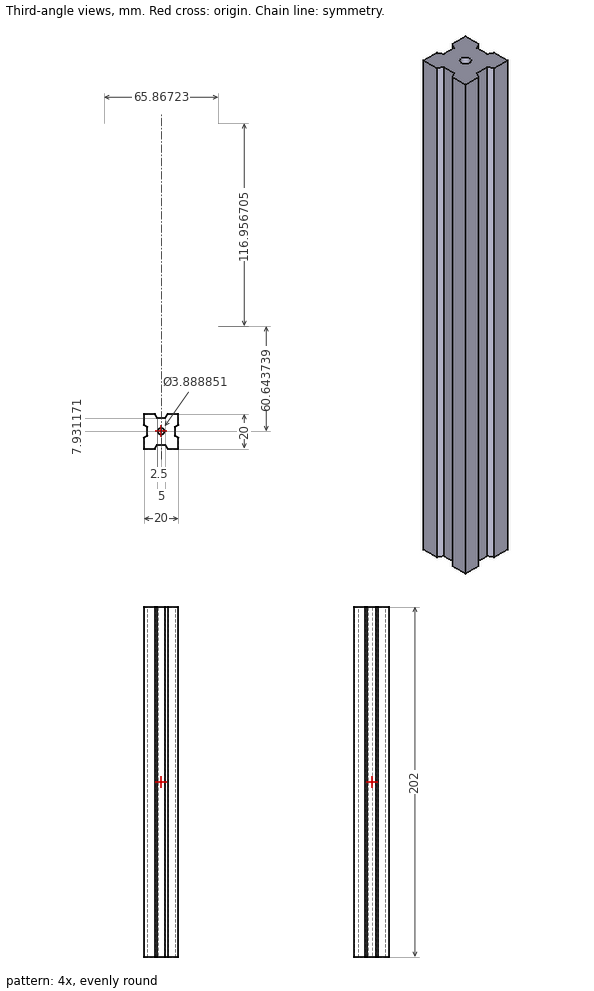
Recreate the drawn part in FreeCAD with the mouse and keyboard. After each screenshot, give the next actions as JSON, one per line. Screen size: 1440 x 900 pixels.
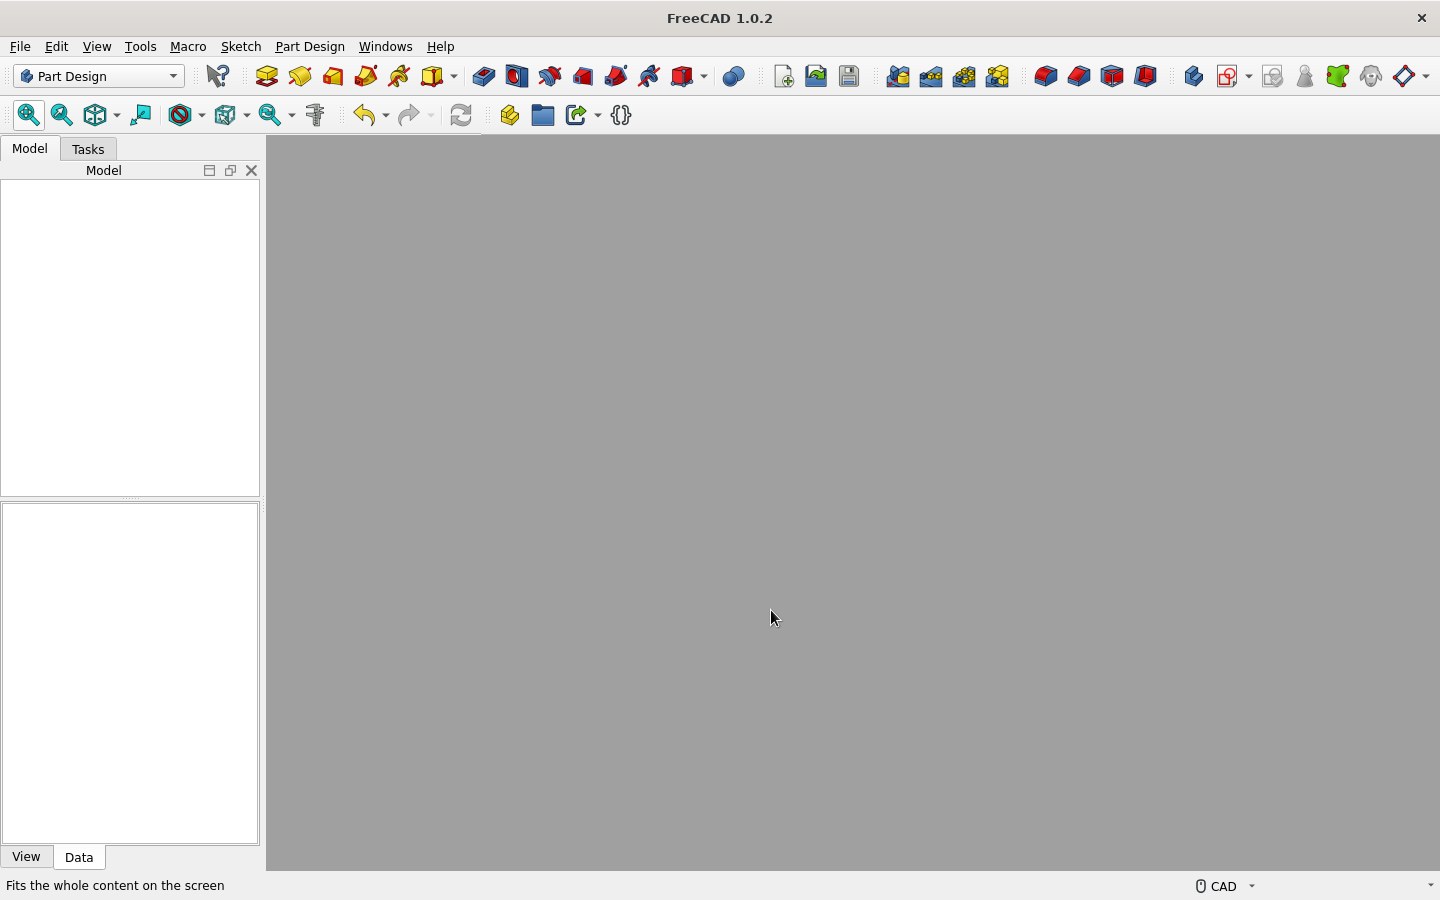
{"action": "key", "text": "ctrl+n"}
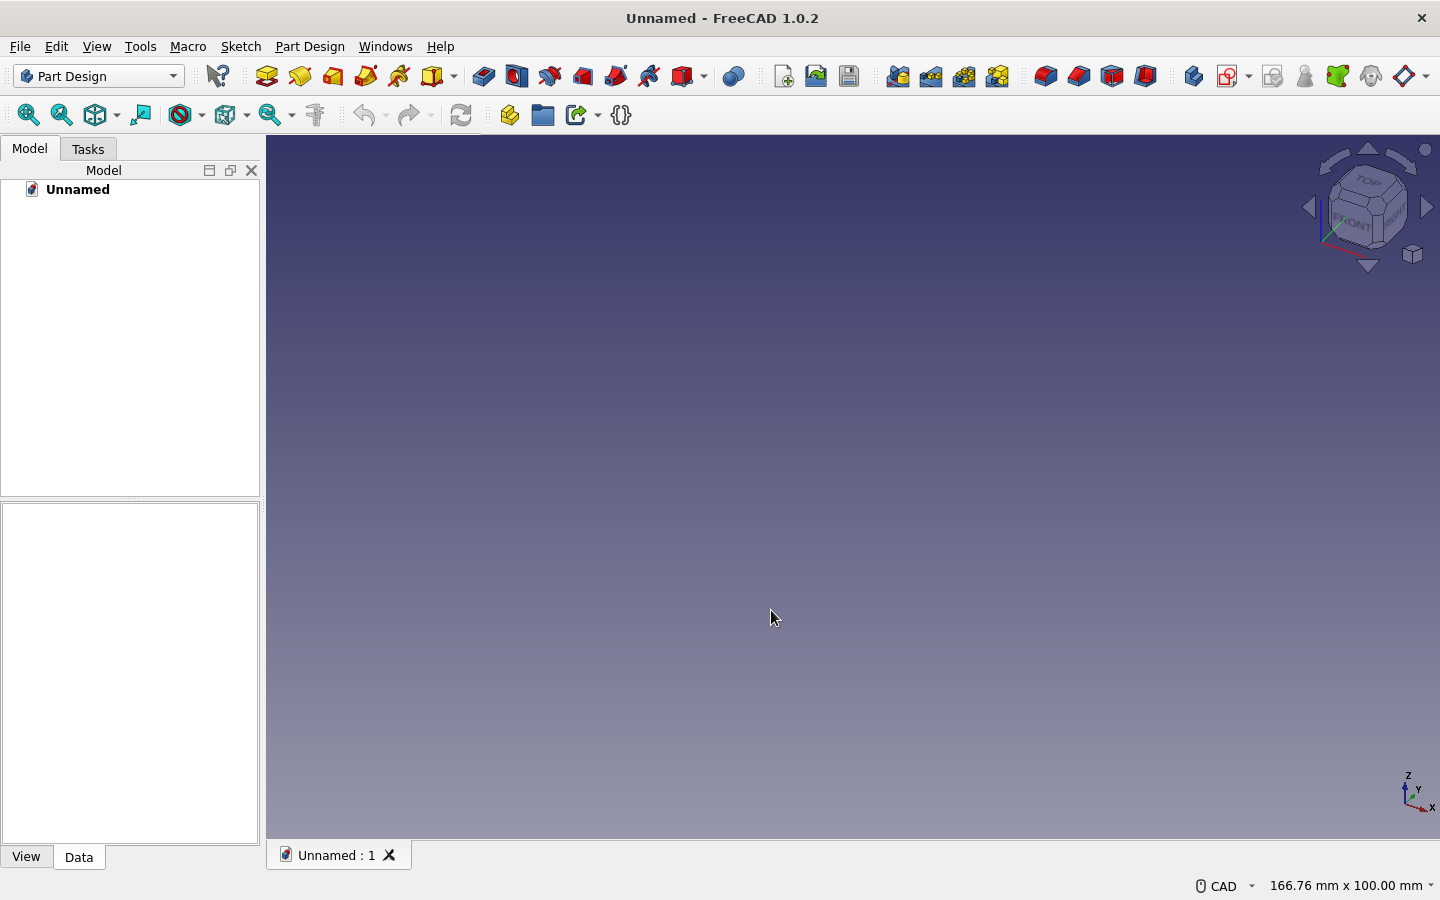
{"action": "left_click", "coordinate": [1226, 76]}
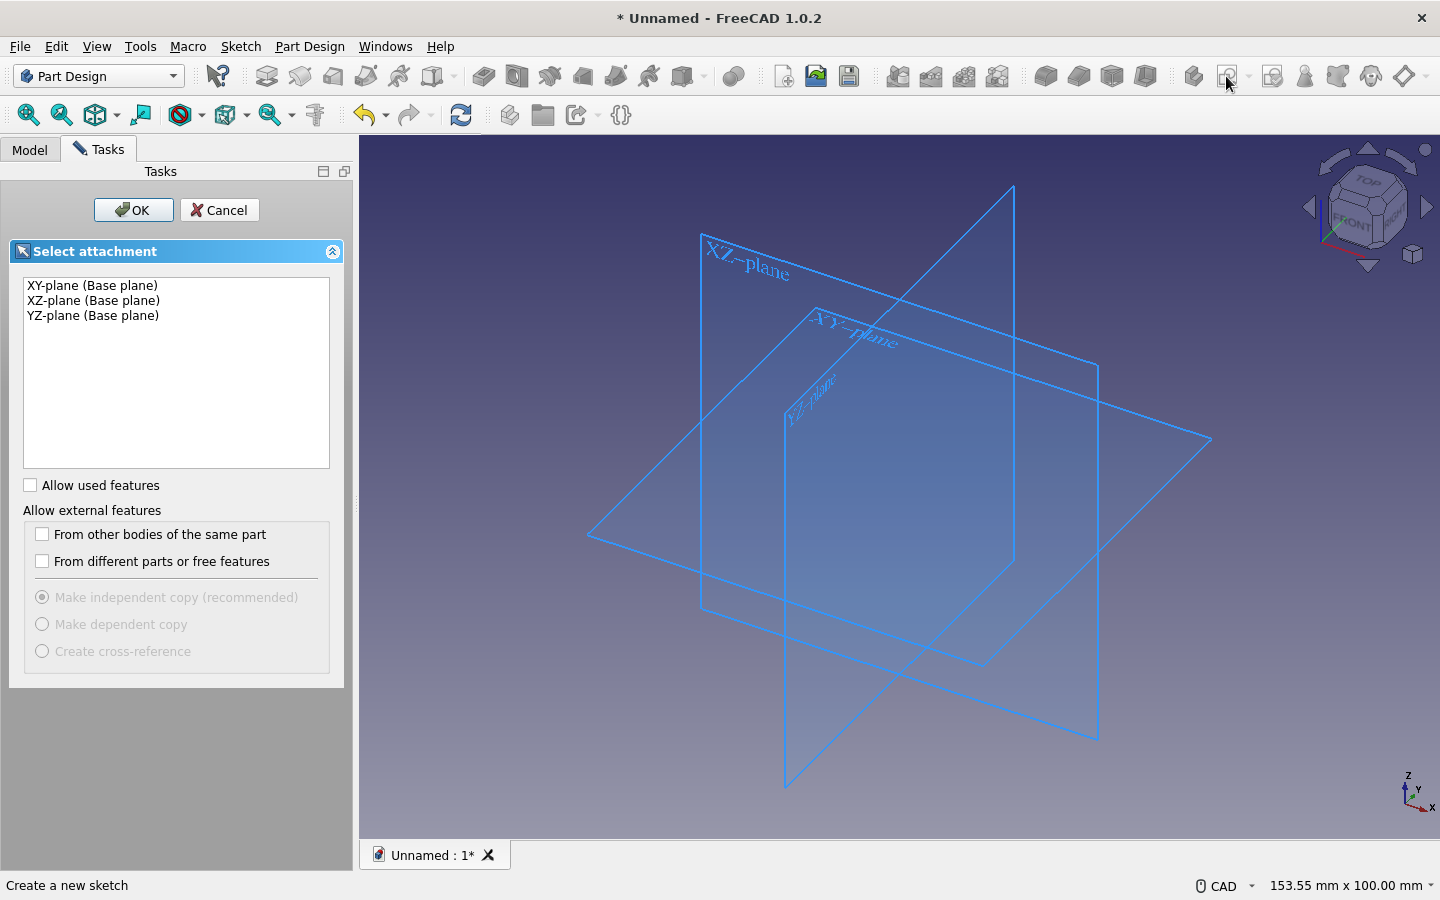
{"action": "left_click", "coordinate": [84, 286]}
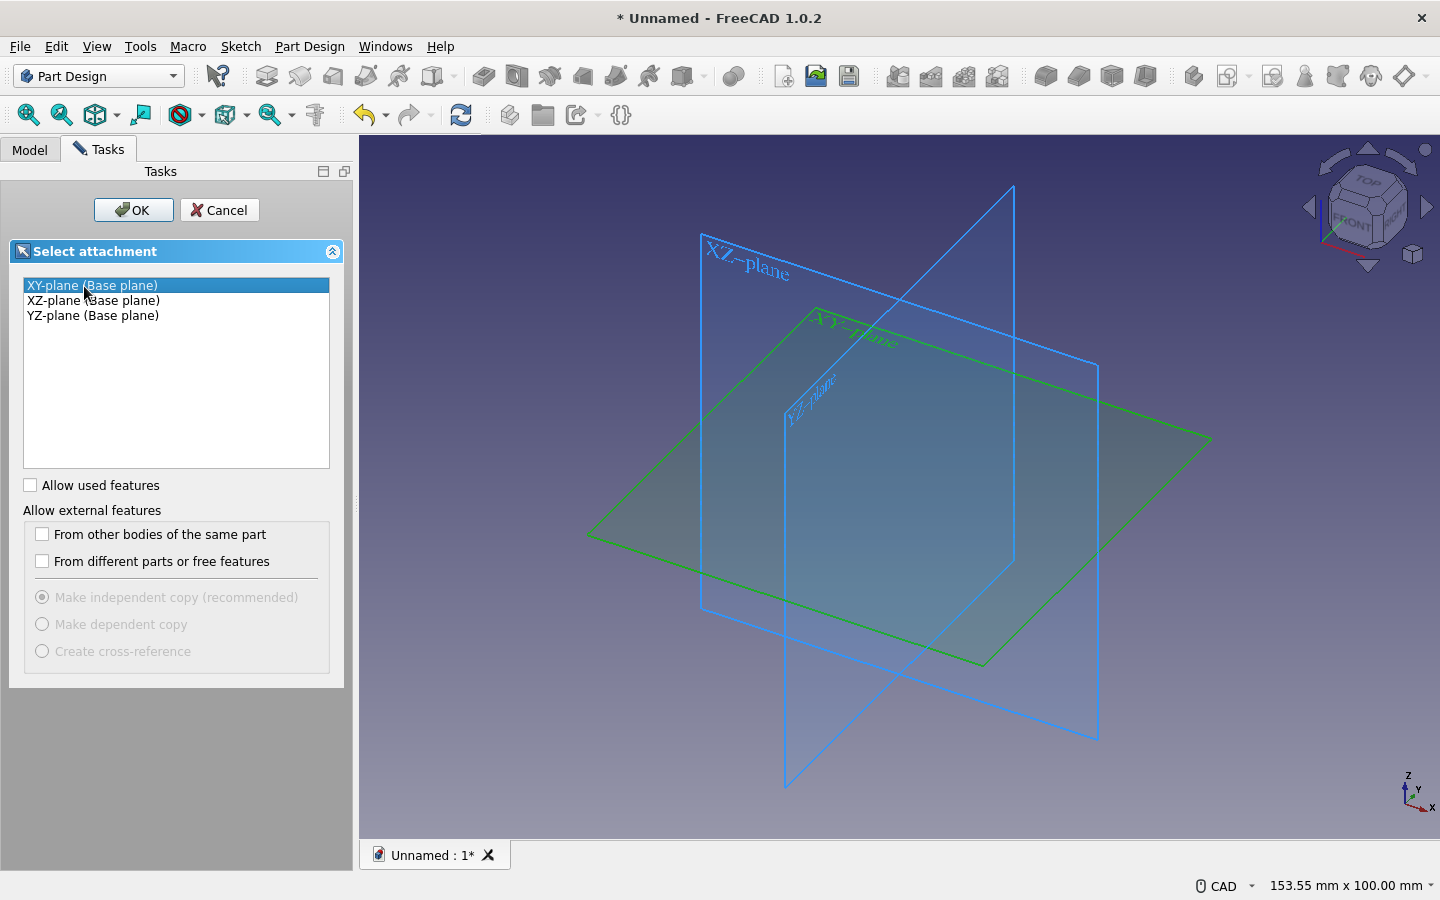
{"action": "left_click", "coordinate": [134, 210]}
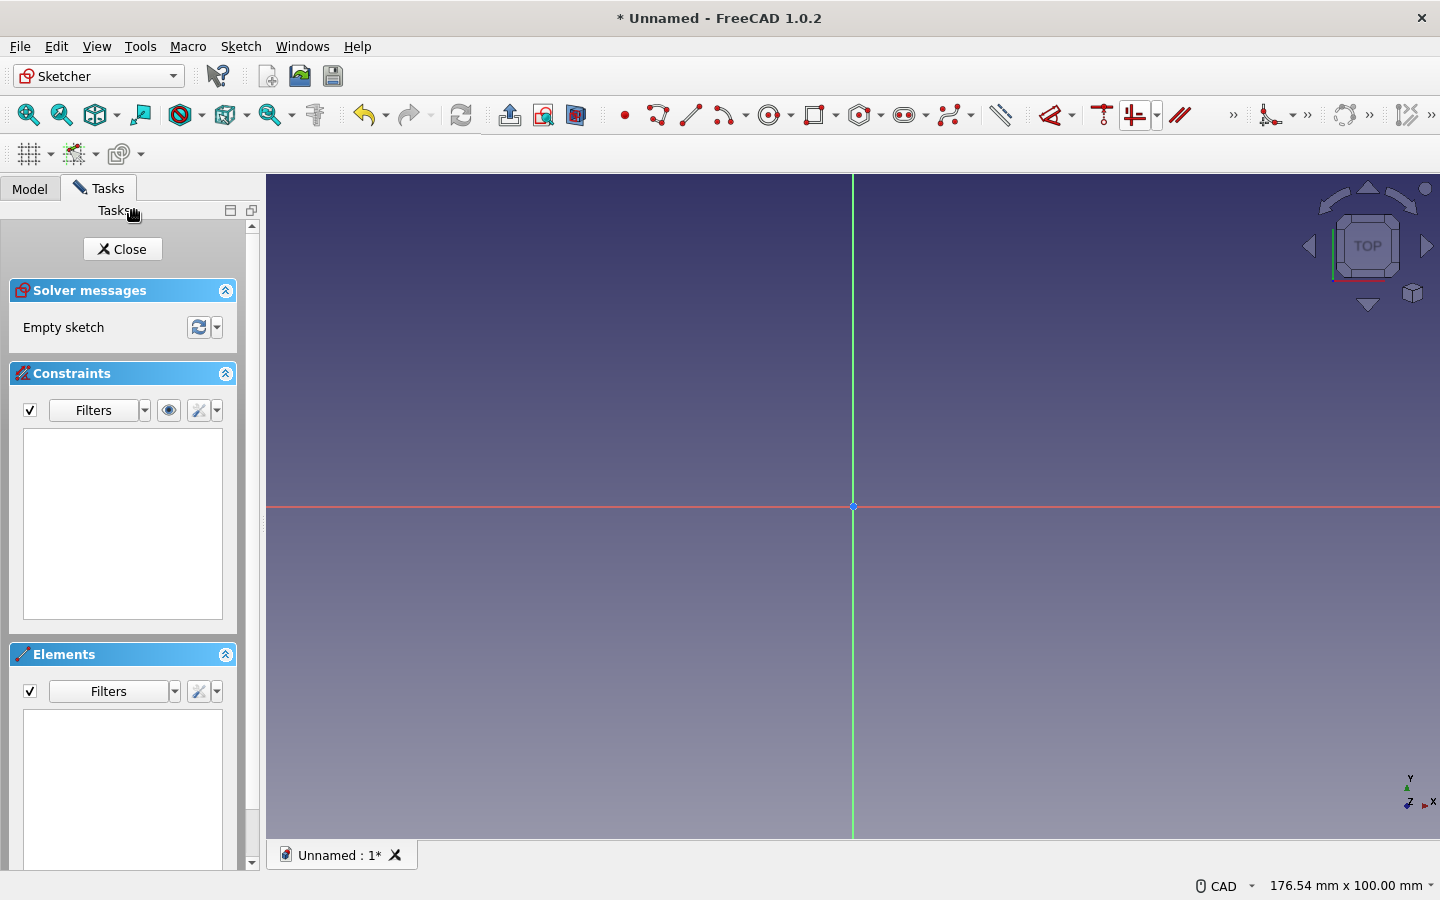
{"action": "scroll", "coordinate": [883, 506], "scroll_direction": "up", "scroll_amount": 6}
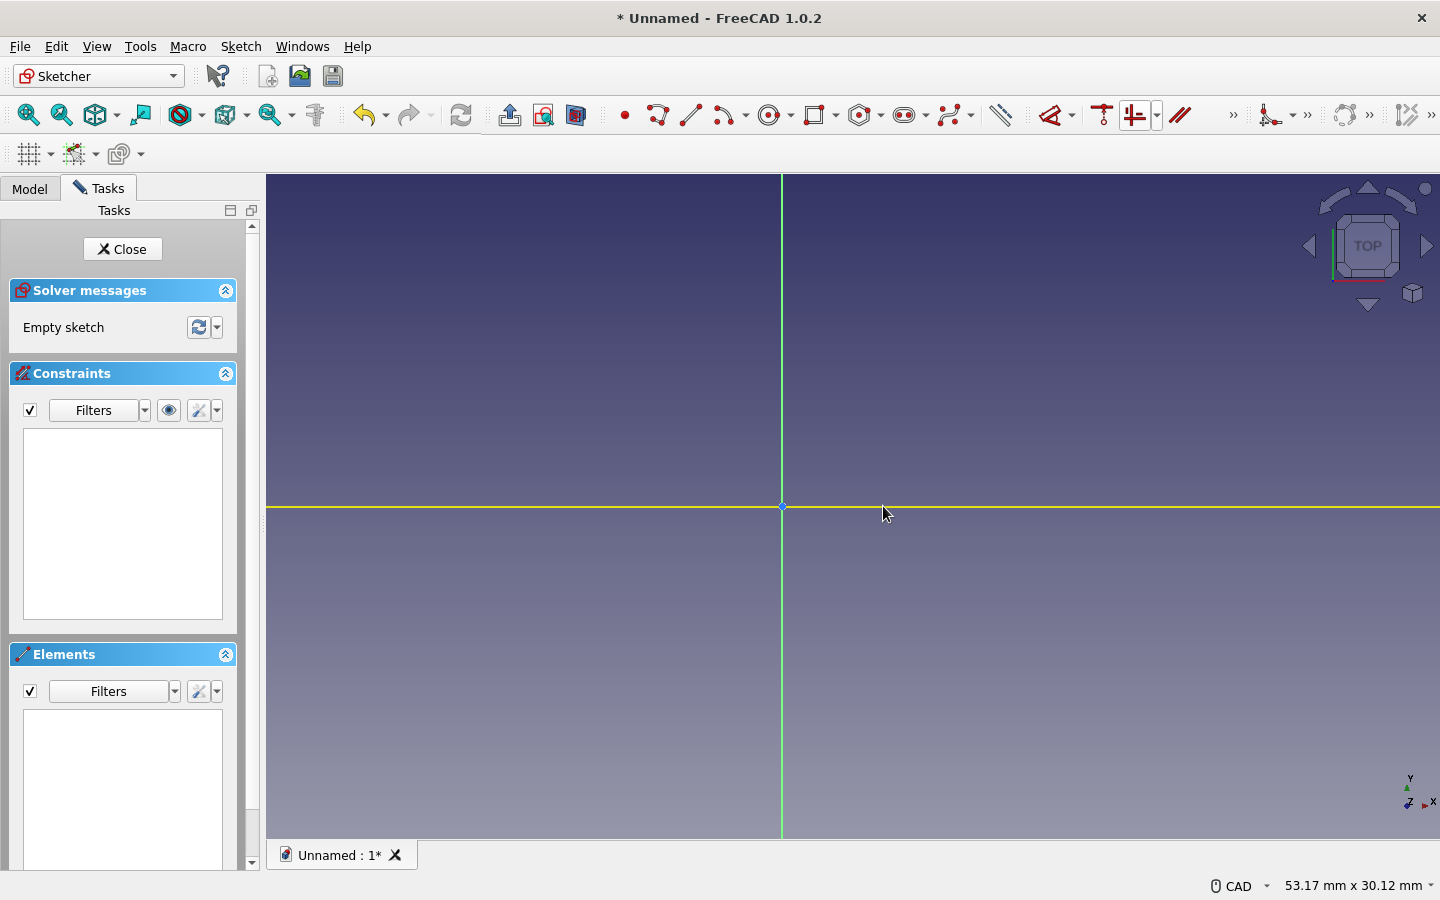
{"action": "key", "text": "g v"}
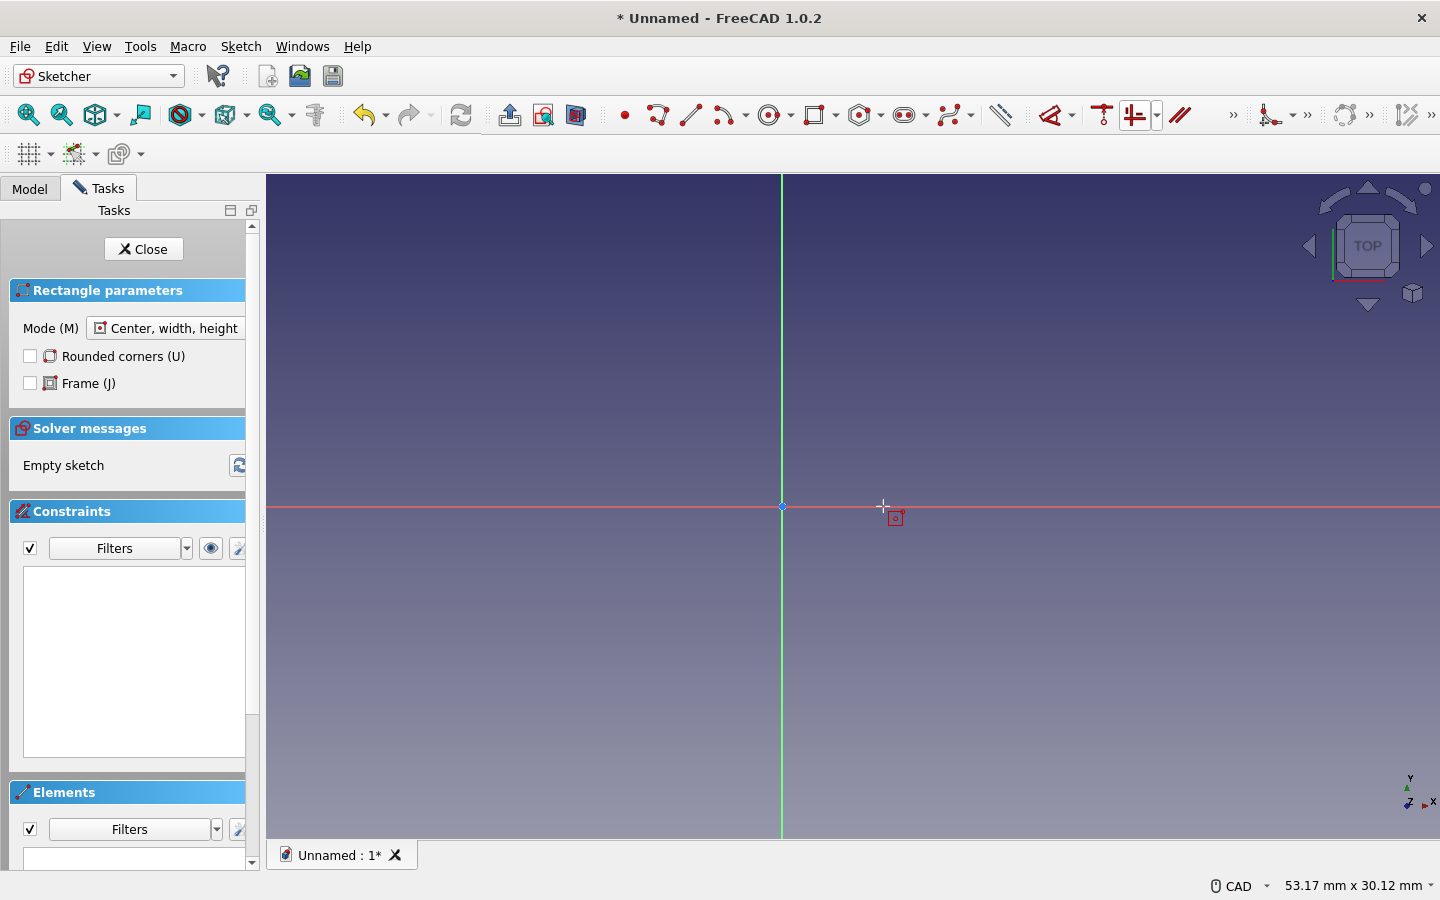
{"action": "left_click", "coordinate": [782, 506]}
{"action": "left_click", "coordinate": [1003, 286]}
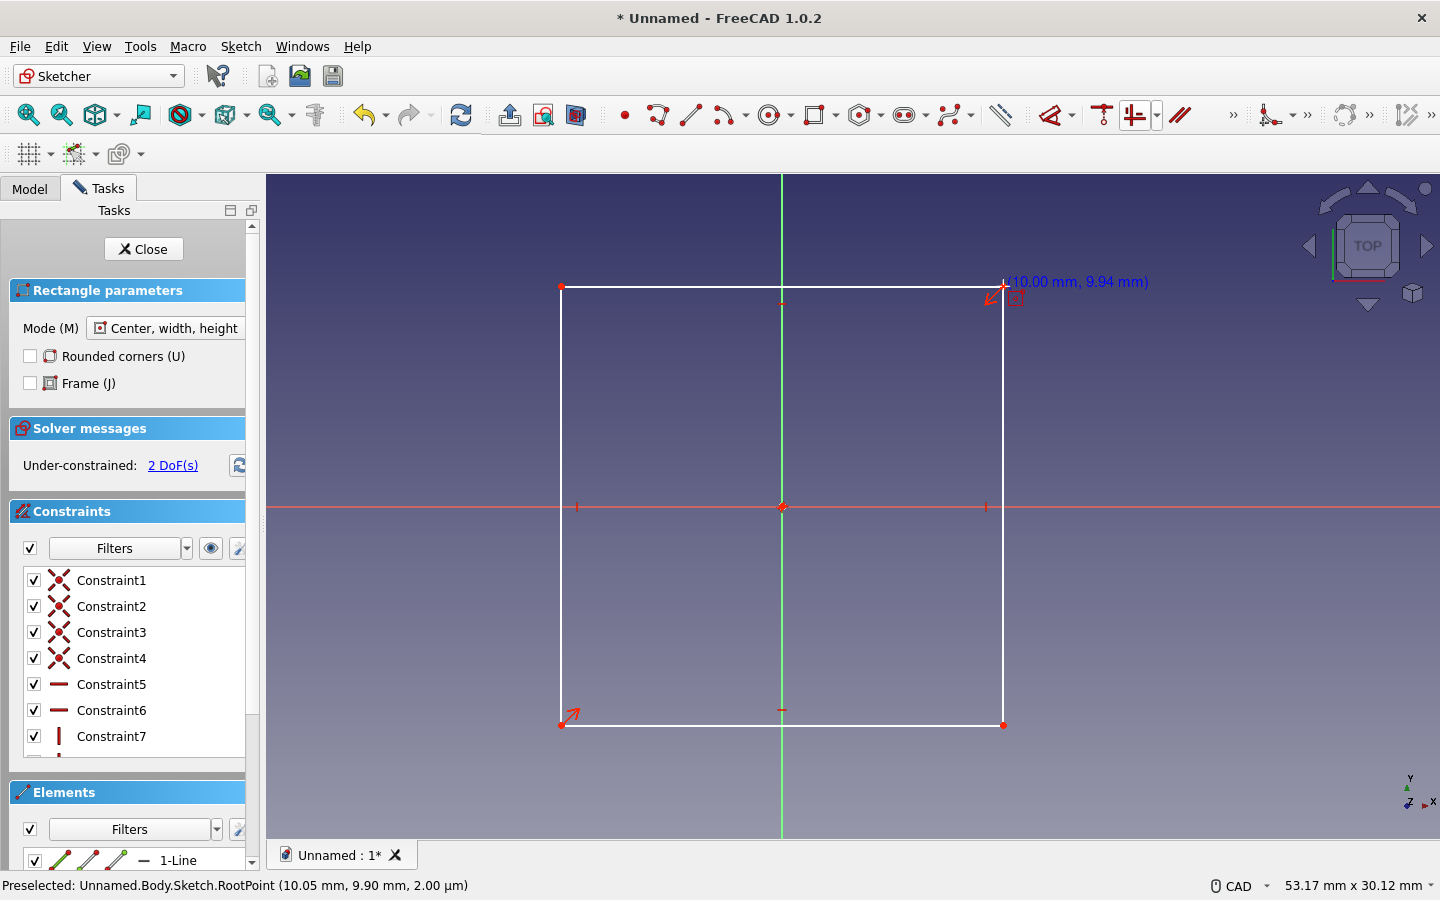
{"action": "key", "text": "g c"}